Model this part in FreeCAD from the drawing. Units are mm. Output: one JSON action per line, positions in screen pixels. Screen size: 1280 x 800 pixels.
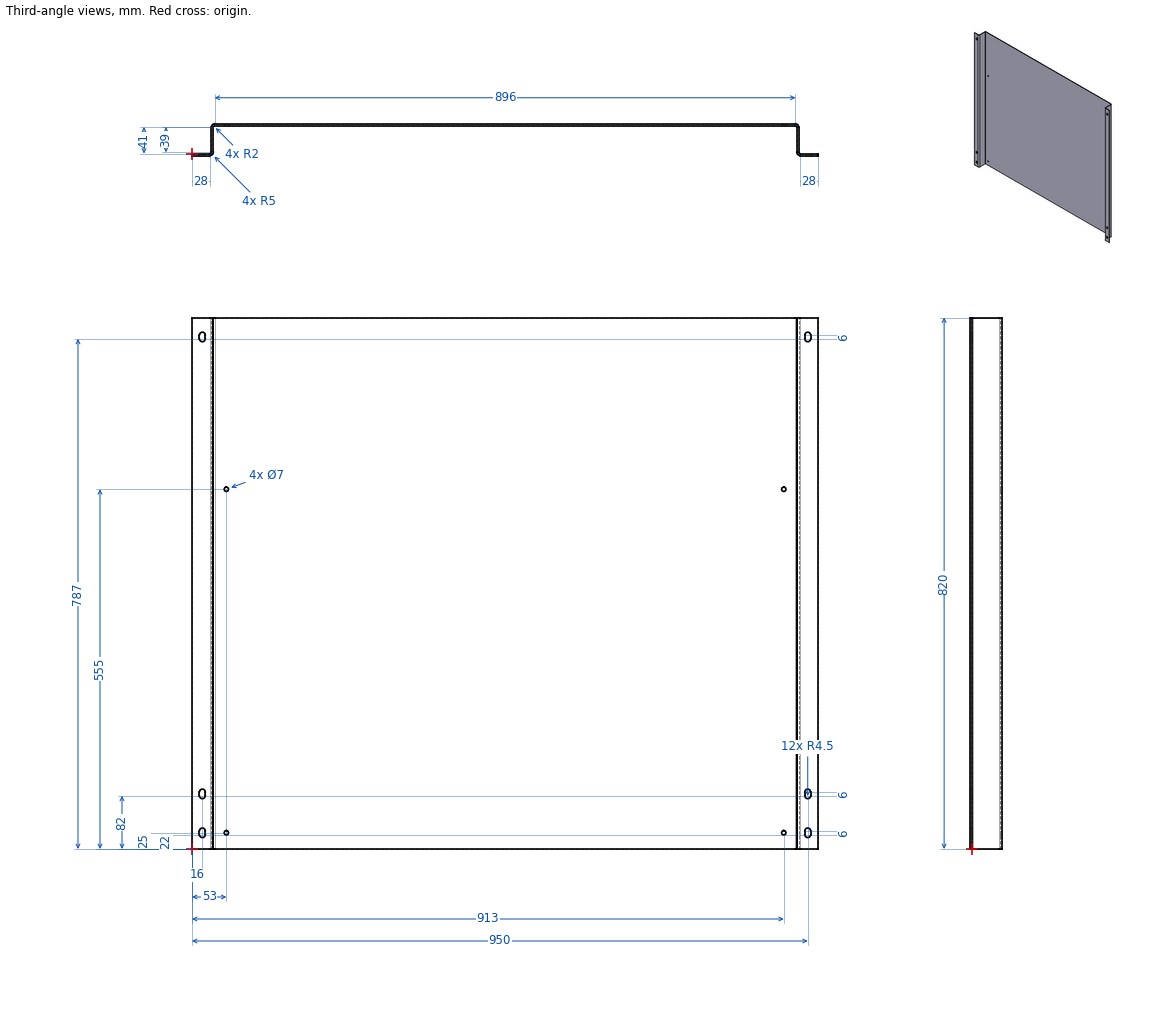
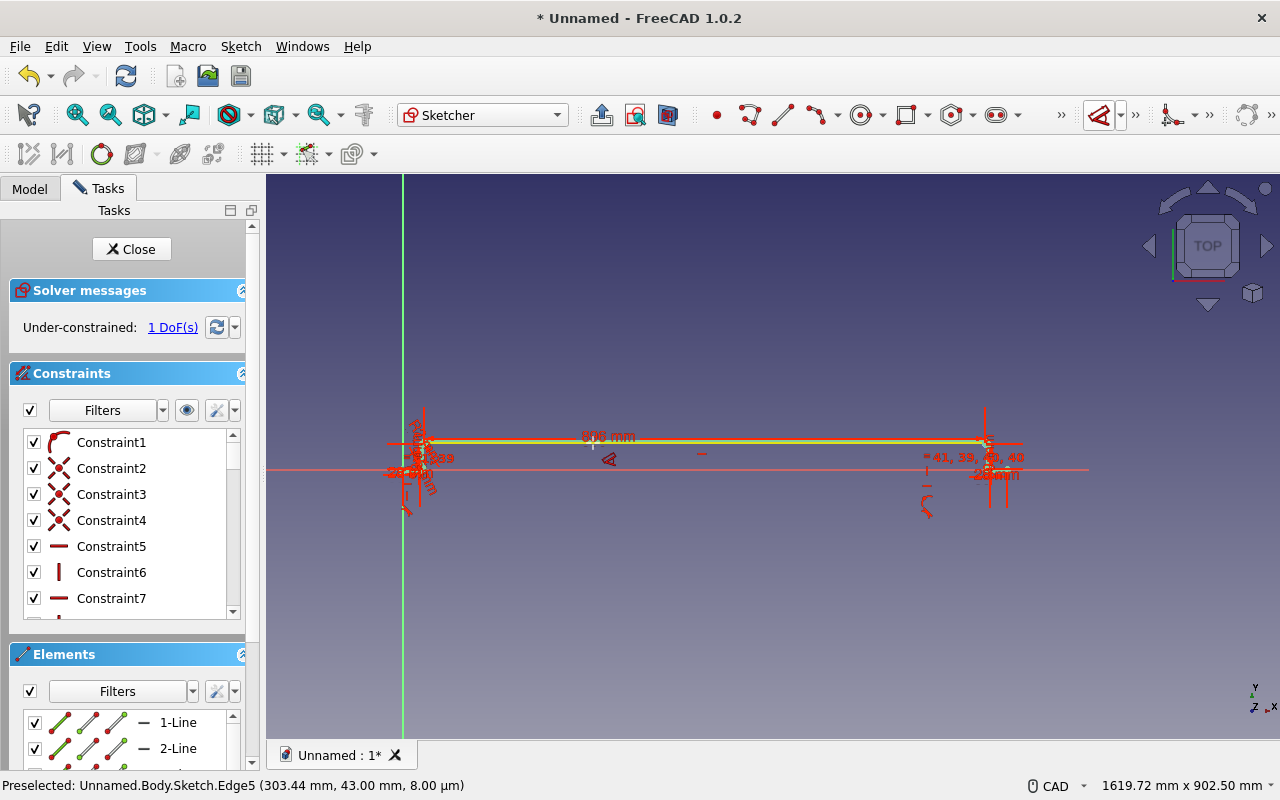
{"action": "scroll", "coordinate": [423, 445], "scroll_direction": "up", "scroll_amount": 12}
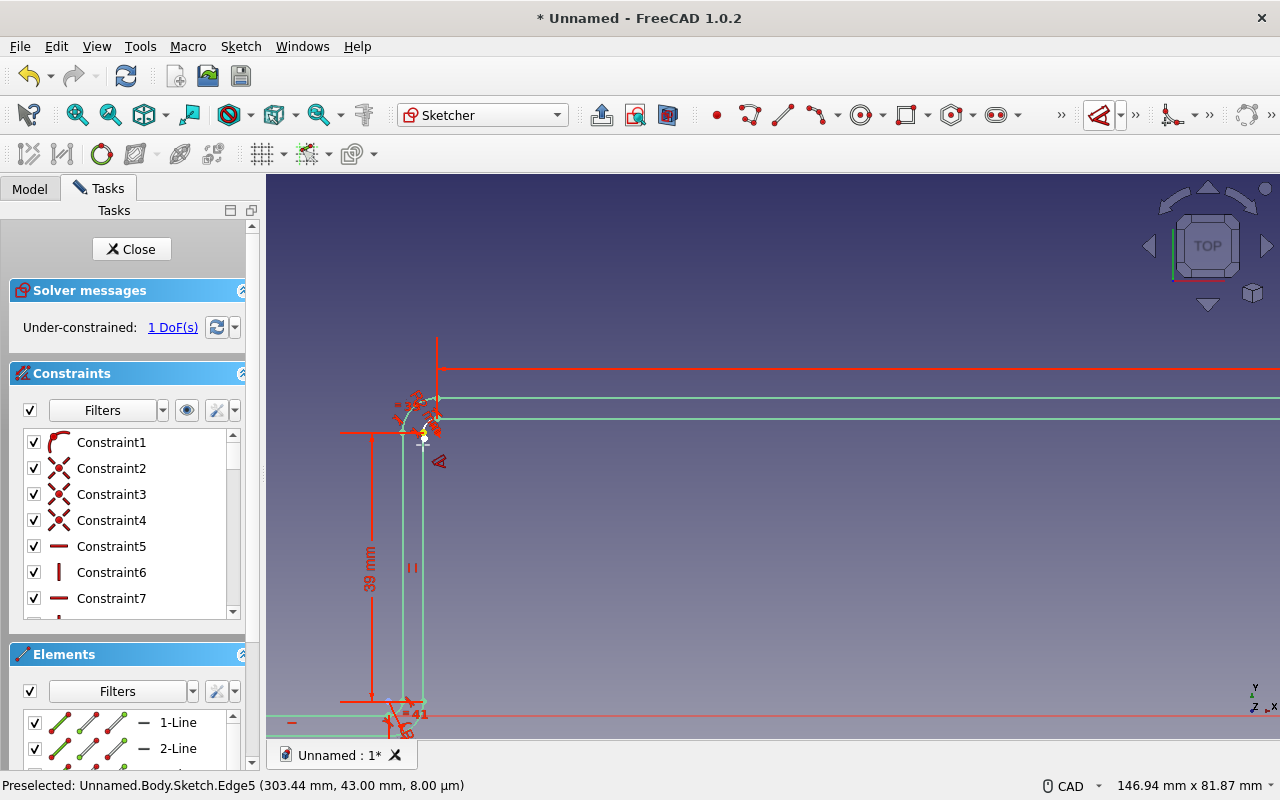
{"action": "left_click", "coordinate": [425, 439]}
{"action": "left_click", "coordinate": [459, 575]}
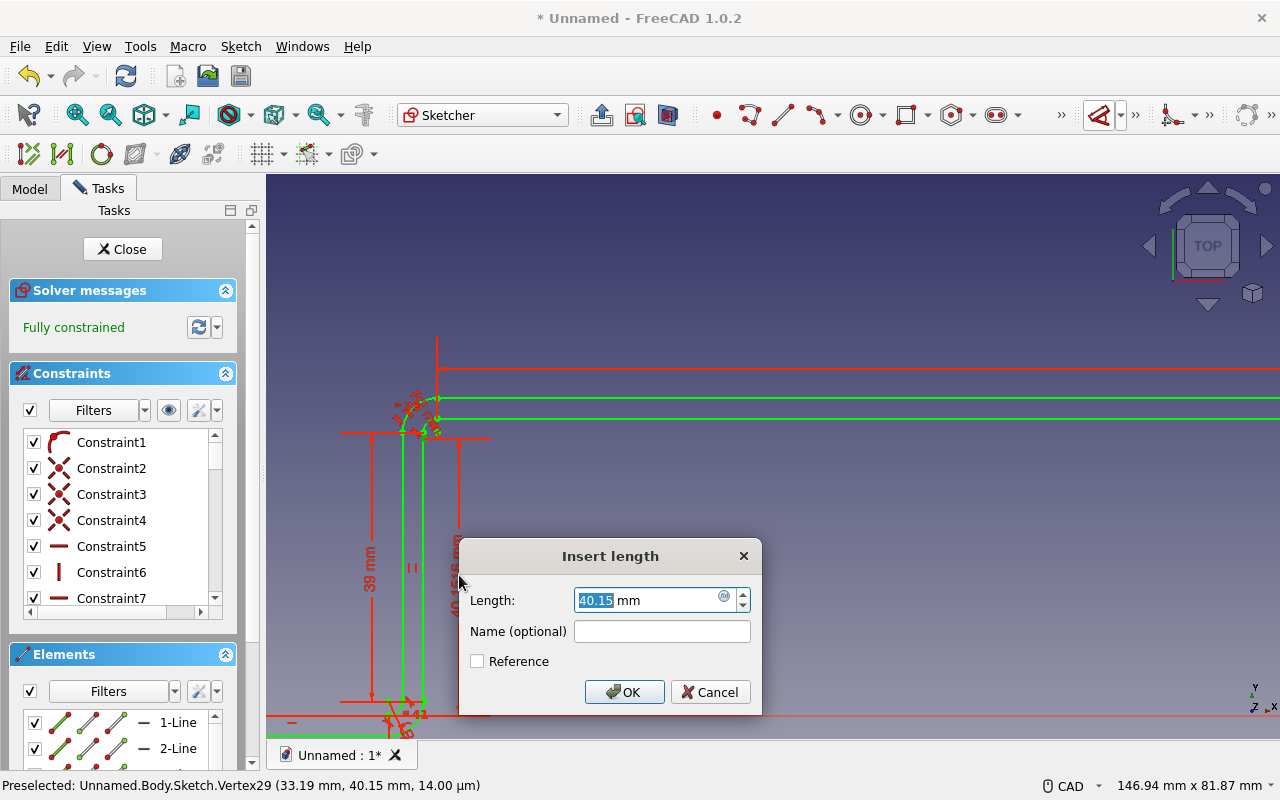
{"action": "type", "text": "41"}
{"action": "key", "text": "Return"}
{"action": "key", "text": "Escape"}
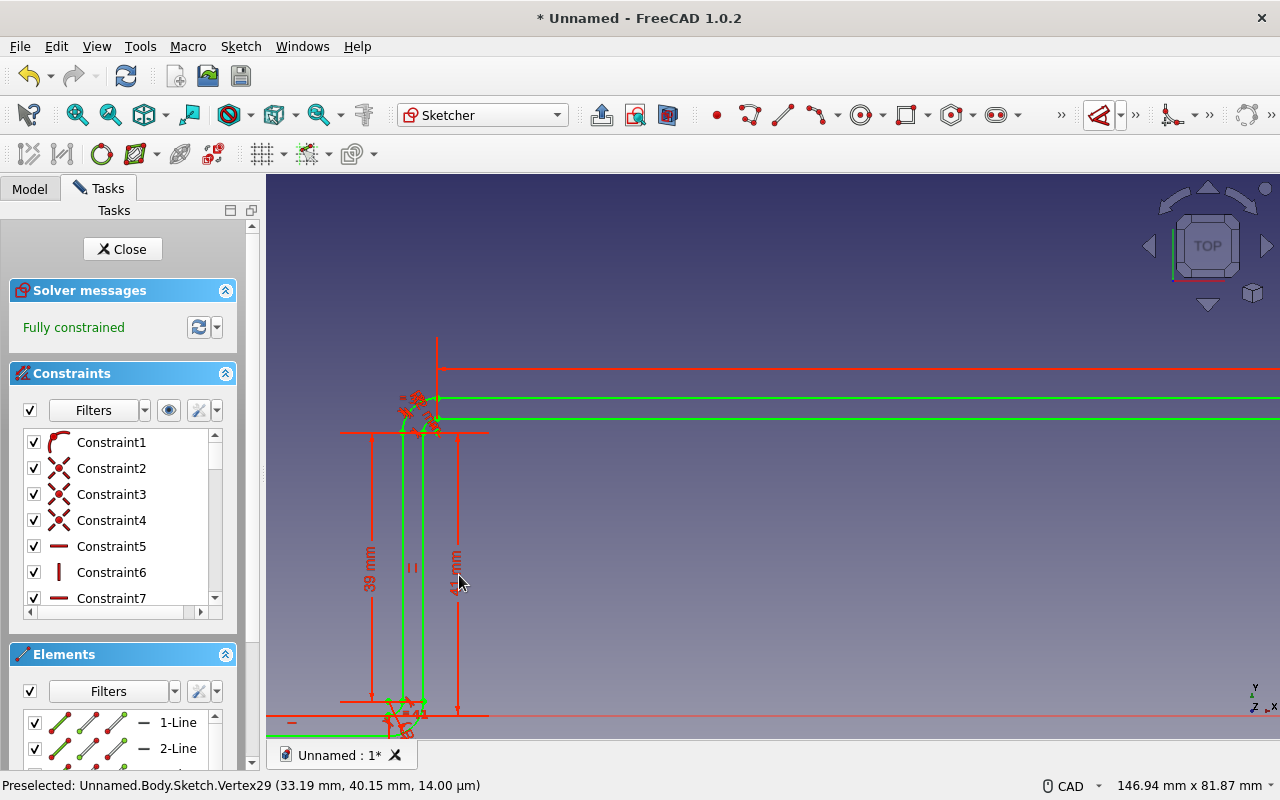
{"action": "left_click", "coordinate": [123, 249]}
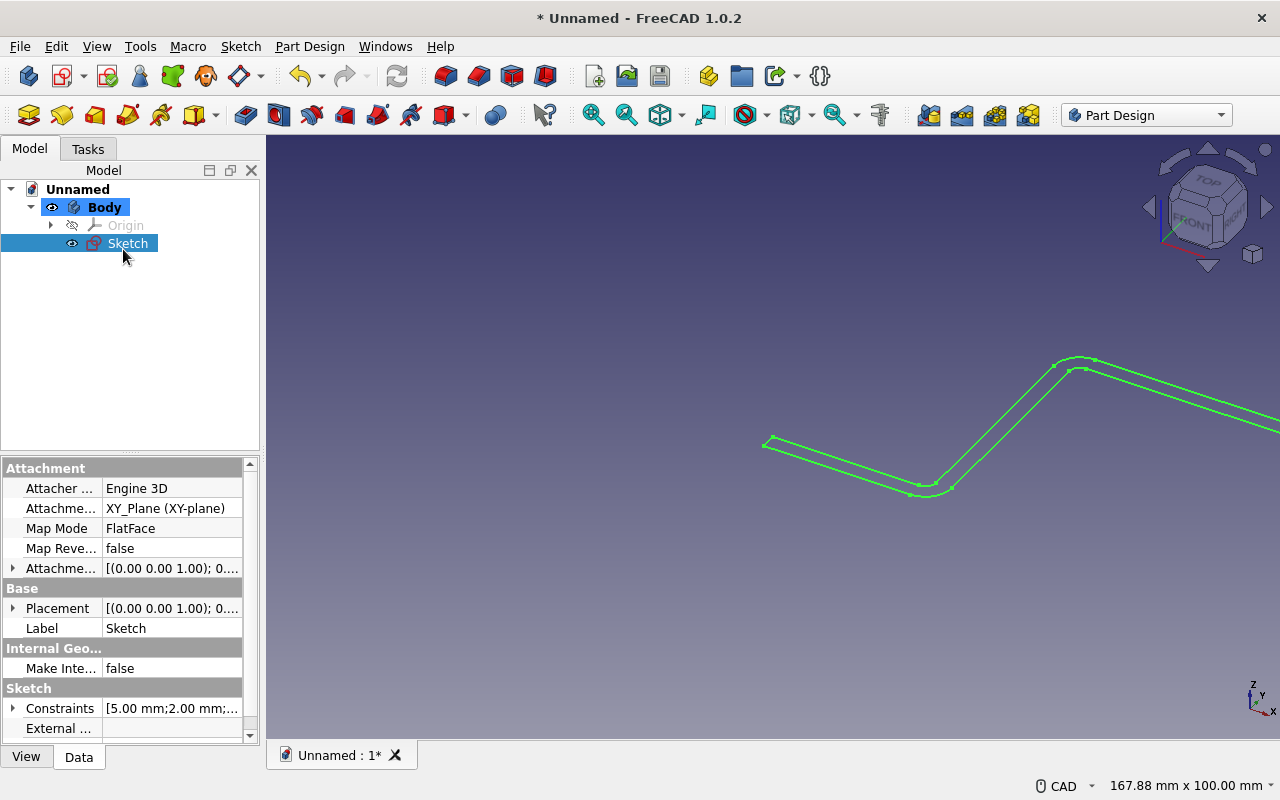
{"action": "left_click", "coordinate": [29, 116]}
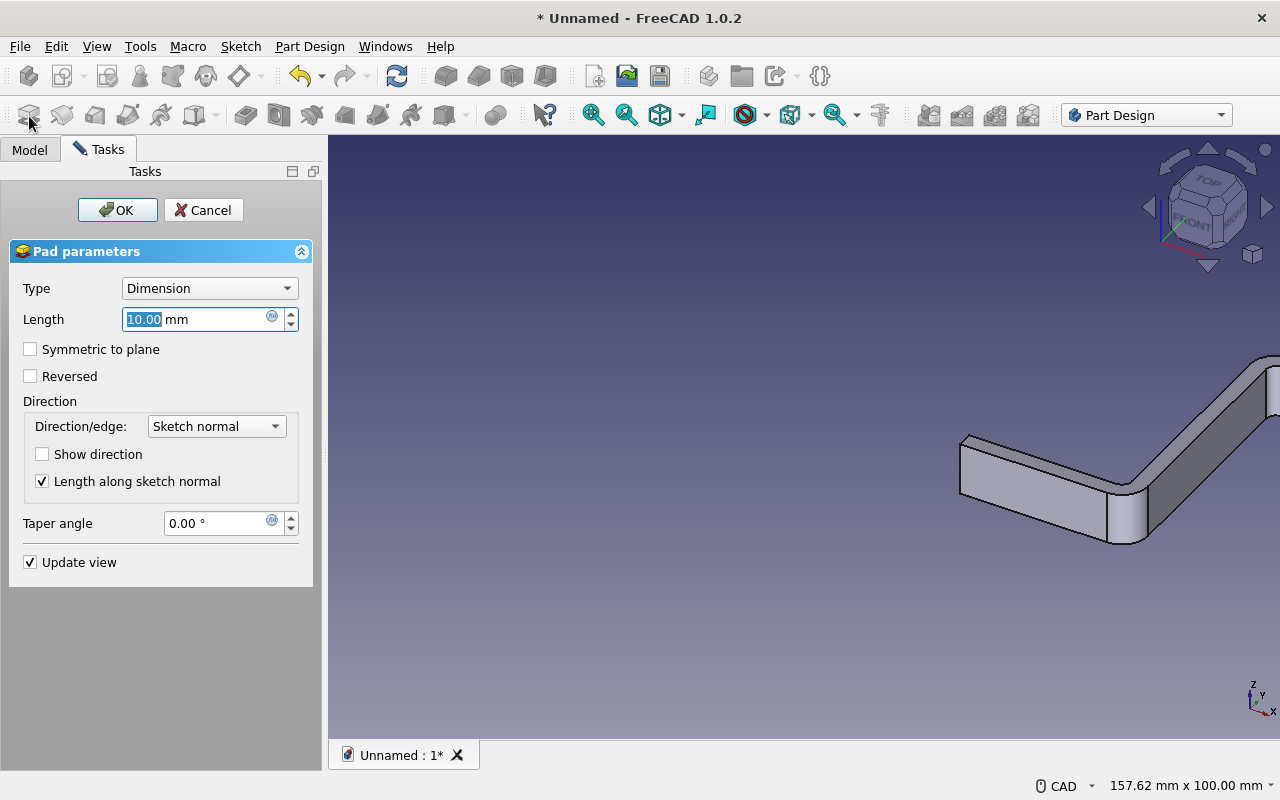
{"action": "type", "text": "820"}
{"action": "key", "text": "Tab"}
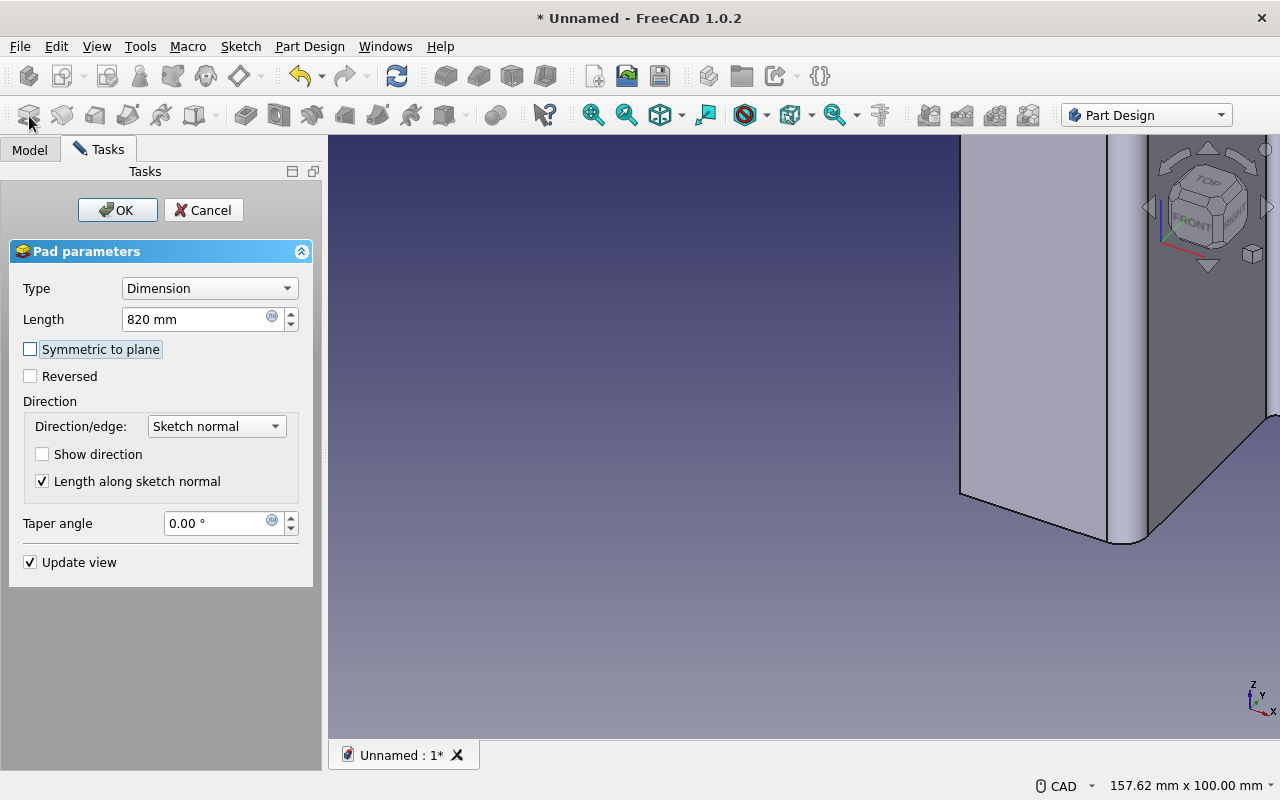
{"action": "left_click", "coordinate": [118, 210]}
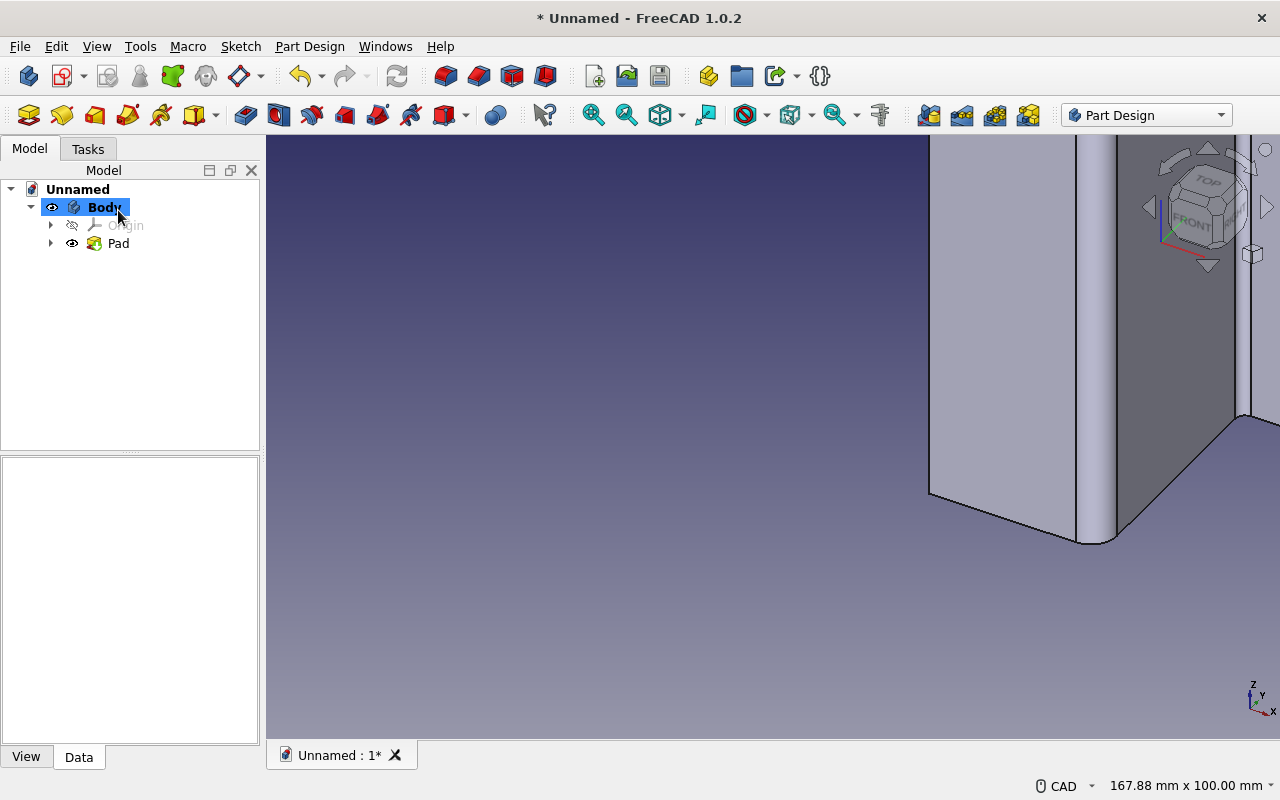
{"action": "left_click", "coordinate": [594, 116]}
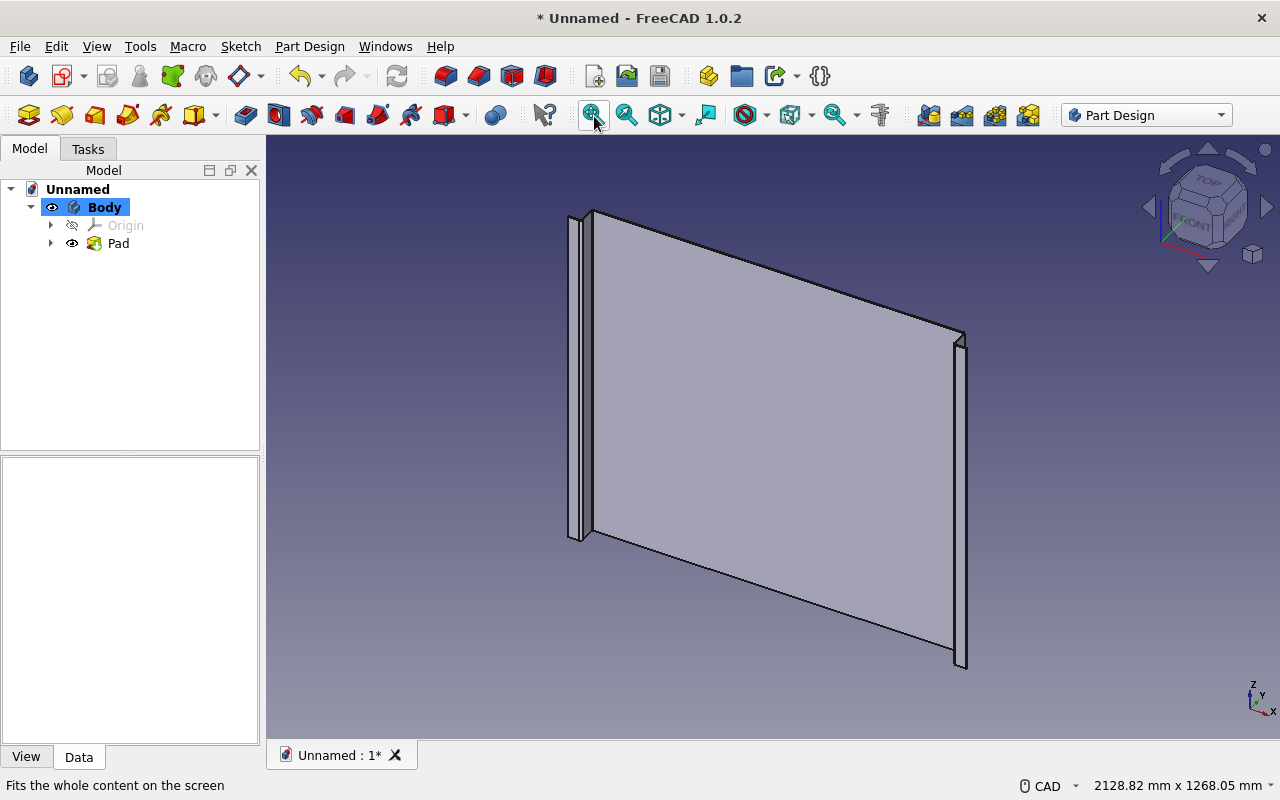
{"action": "key", "text": "4"}